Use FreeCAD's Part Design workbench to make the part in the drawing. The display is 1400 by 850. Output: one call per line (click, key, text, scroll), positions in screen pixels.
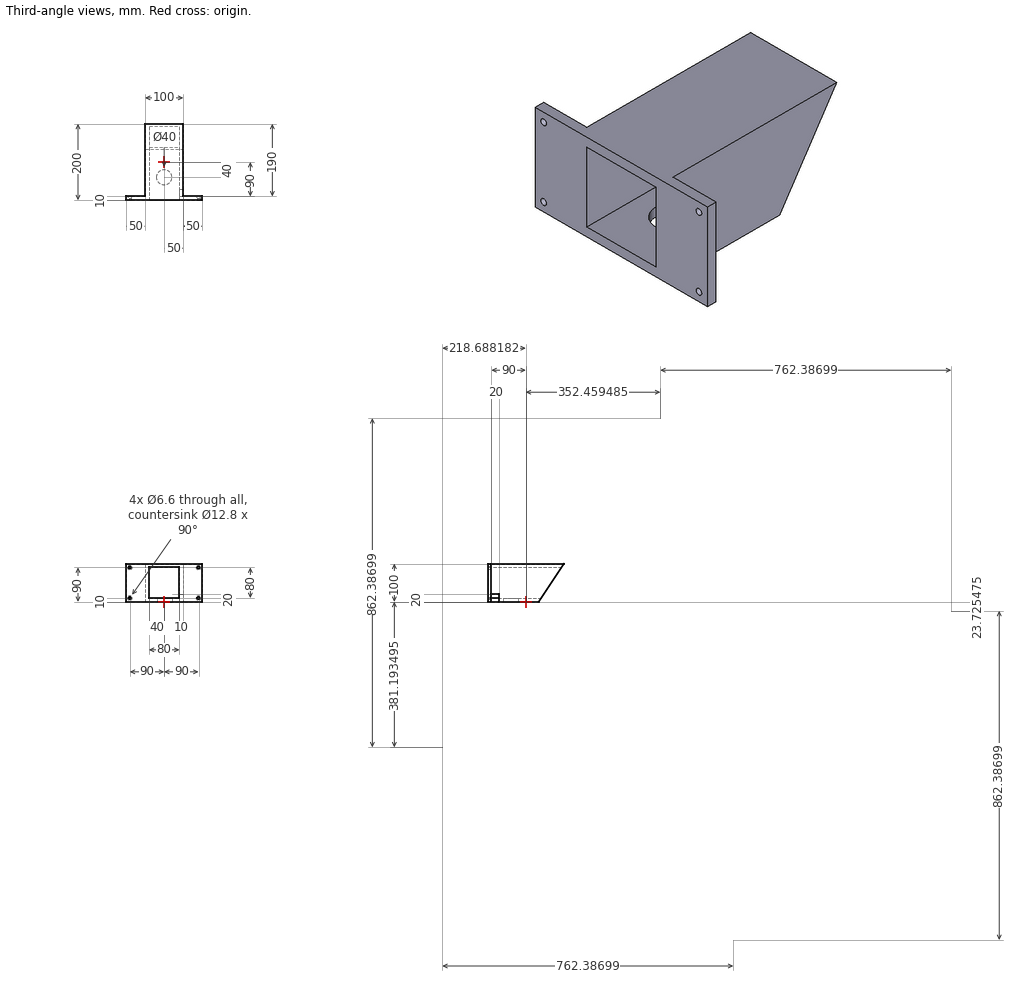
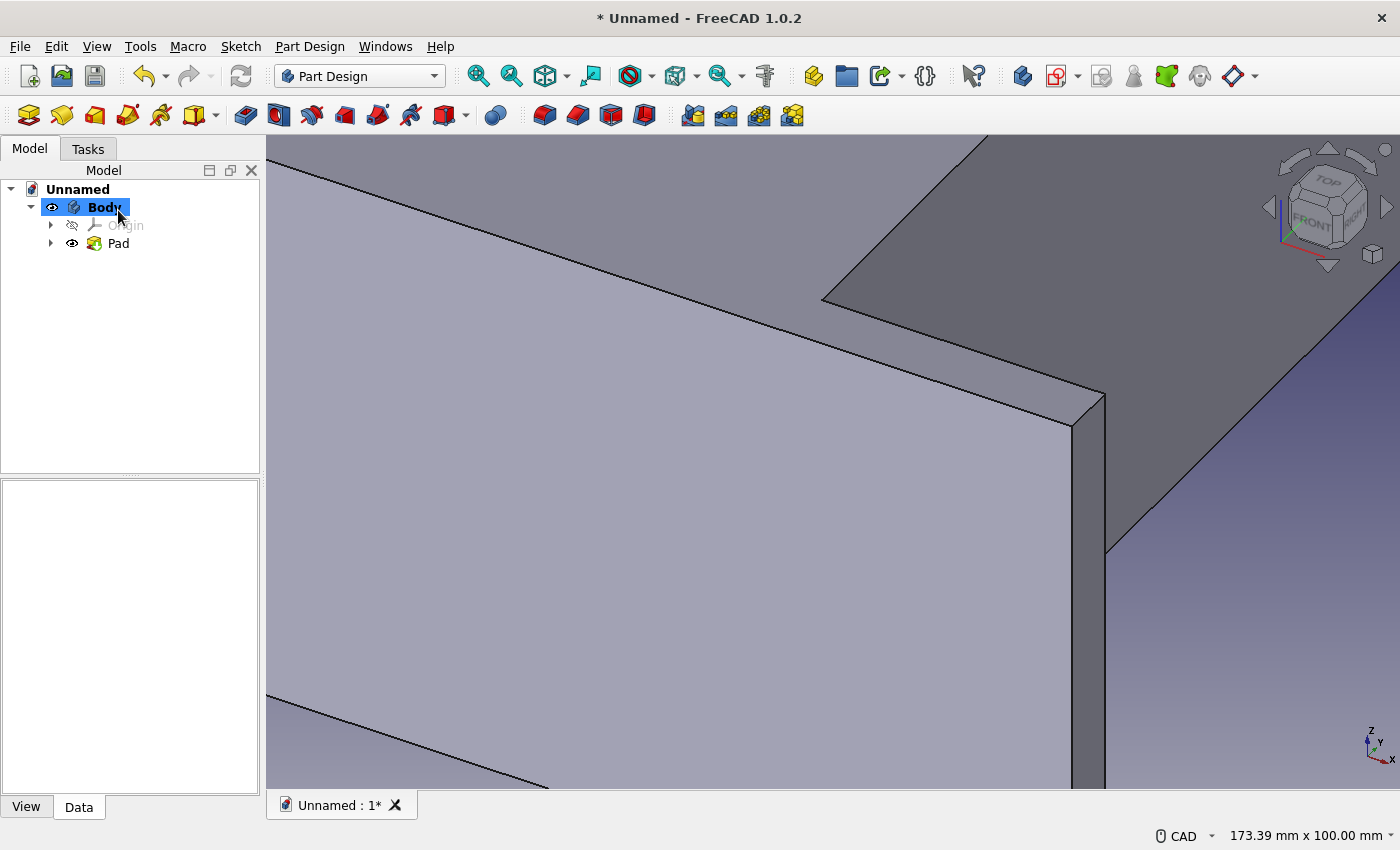
key(v)
key(f)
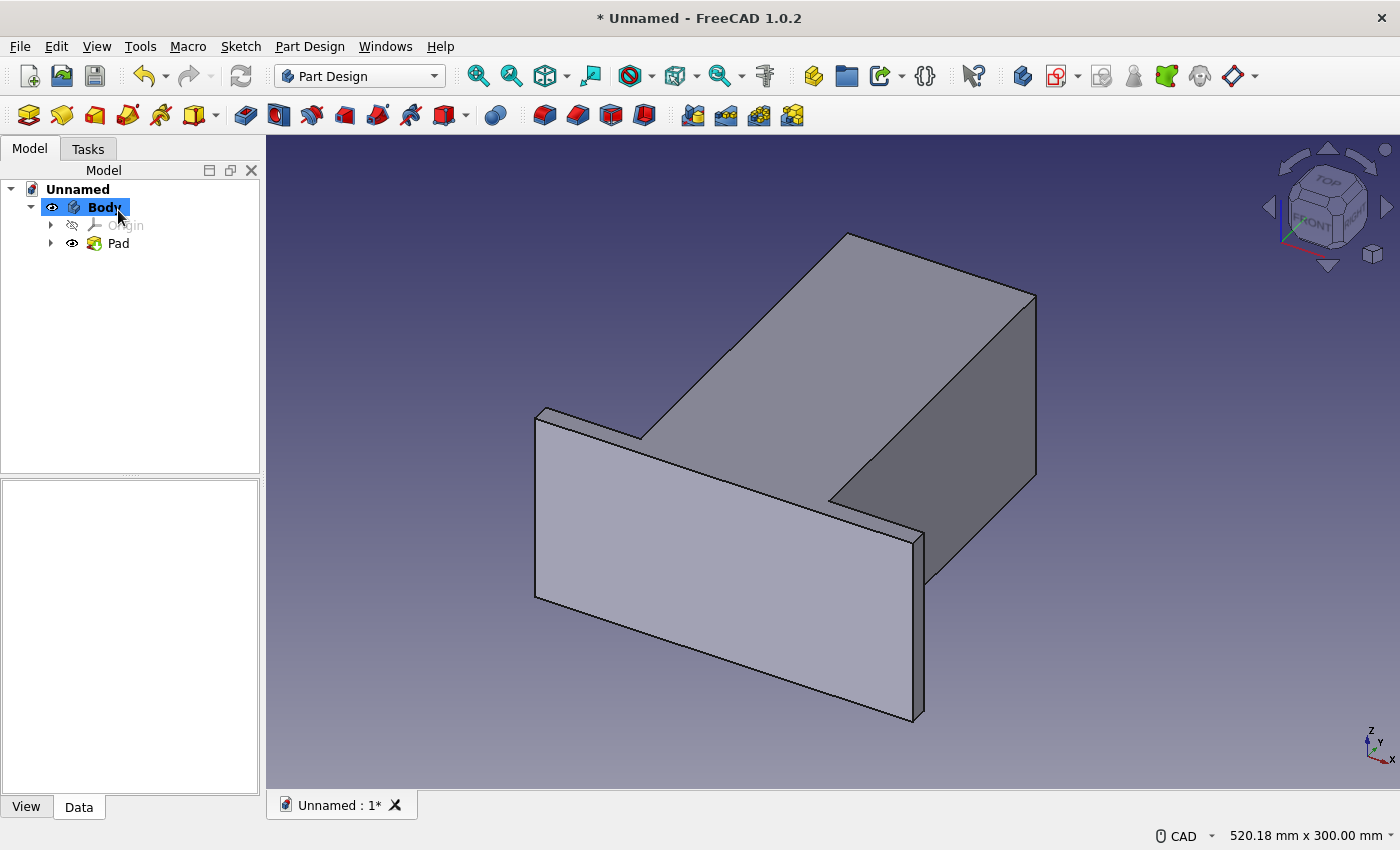
click(1056, 76)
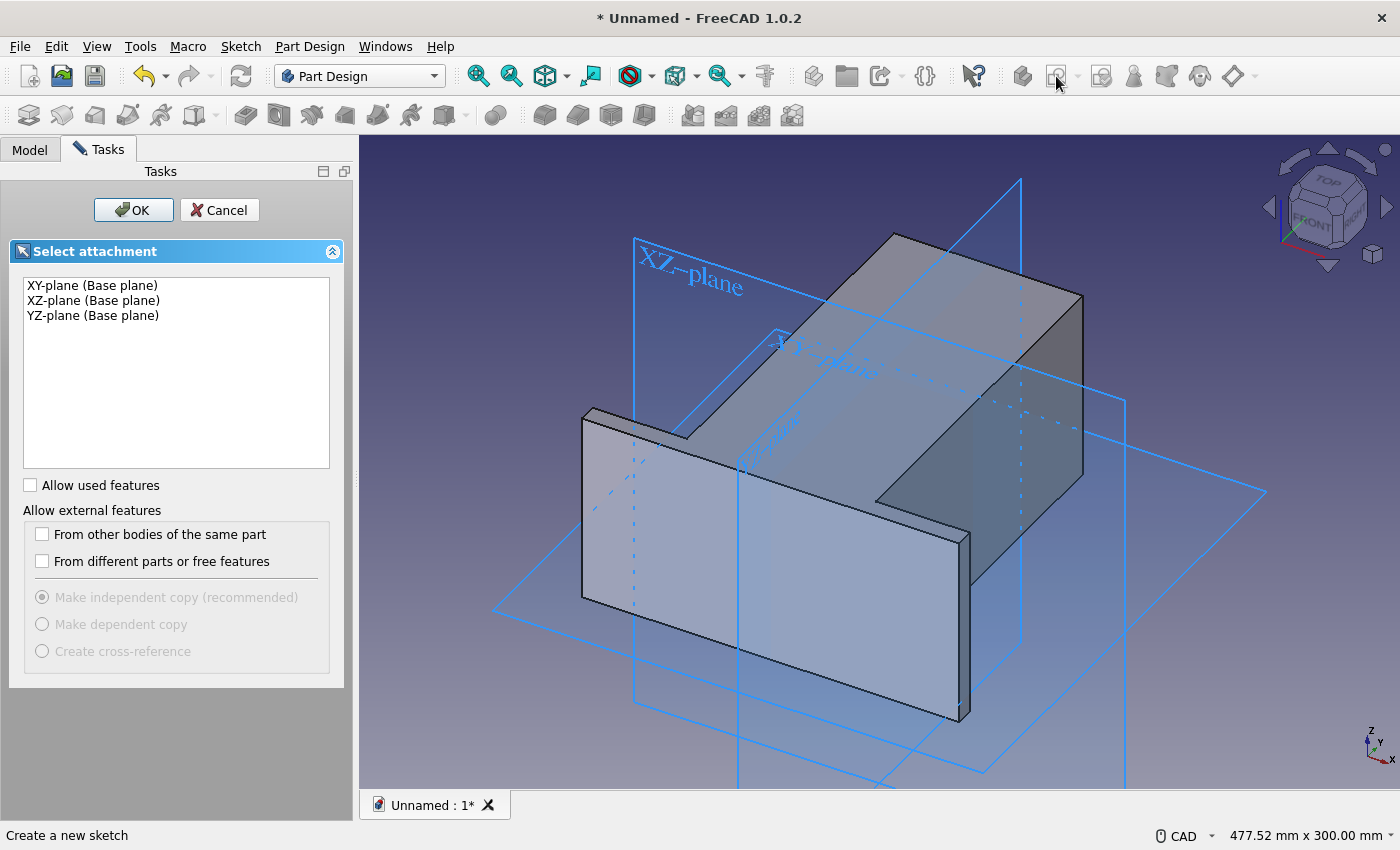
click(84, 316)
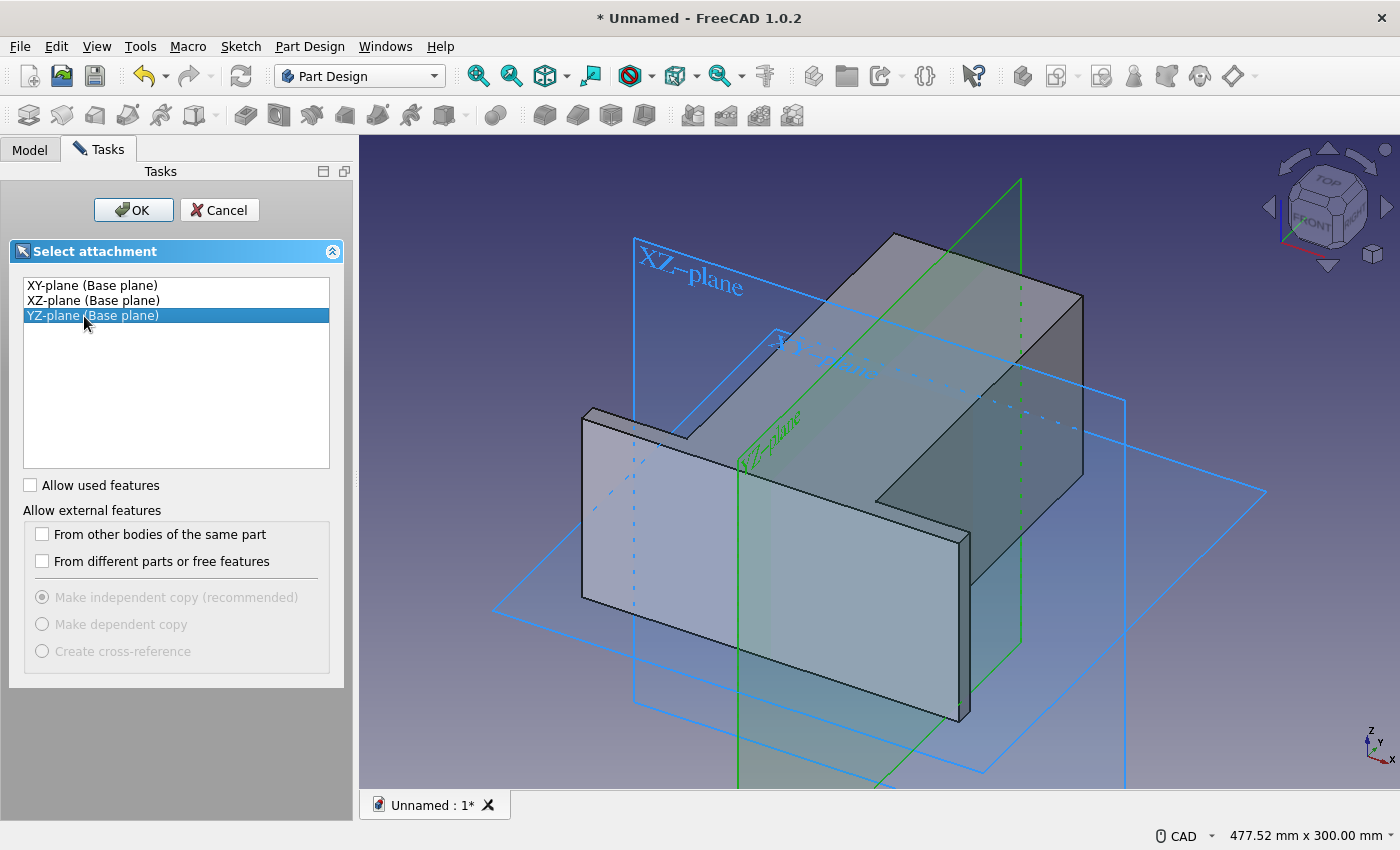
click(134, 210)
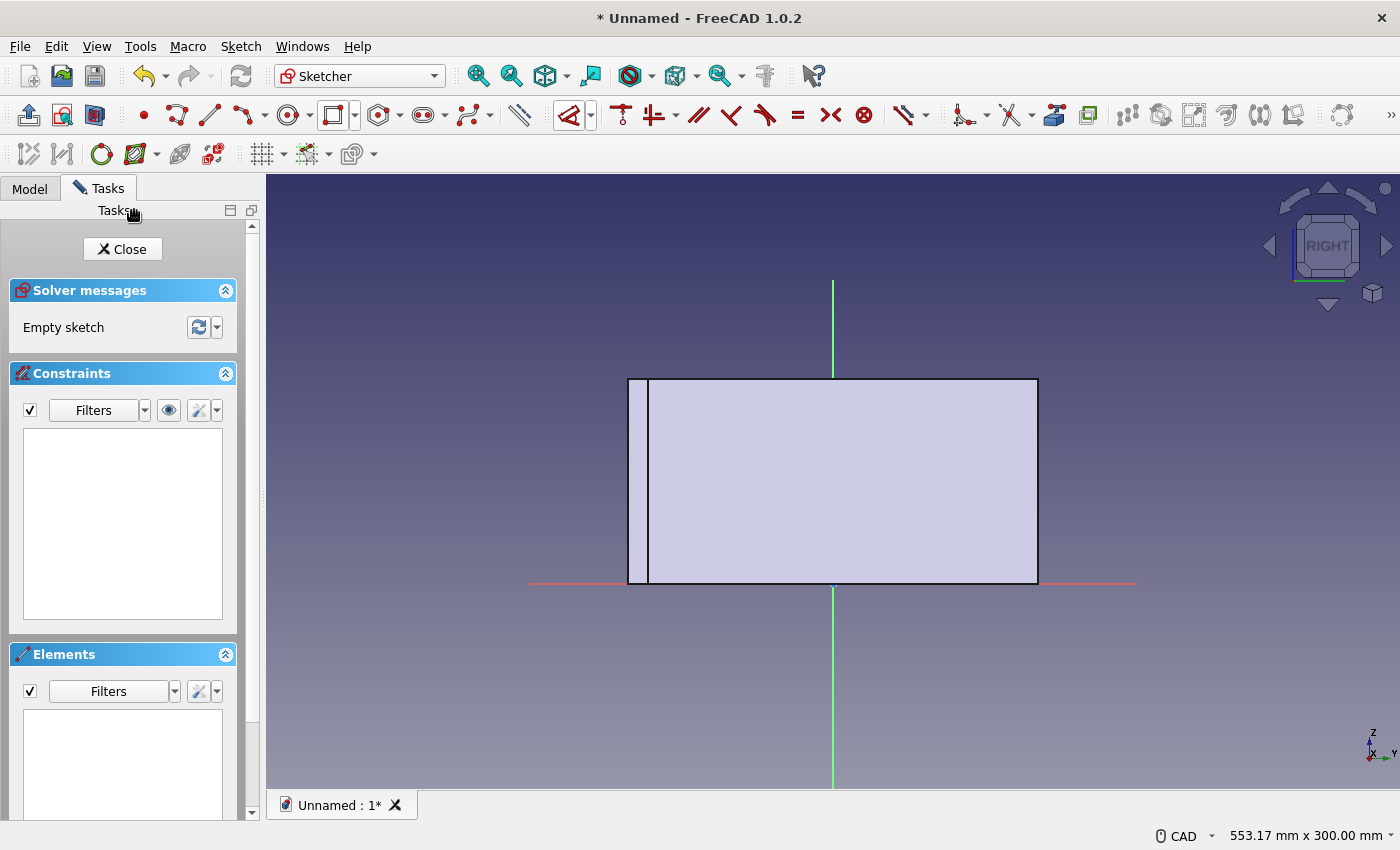
key(q)
key(s)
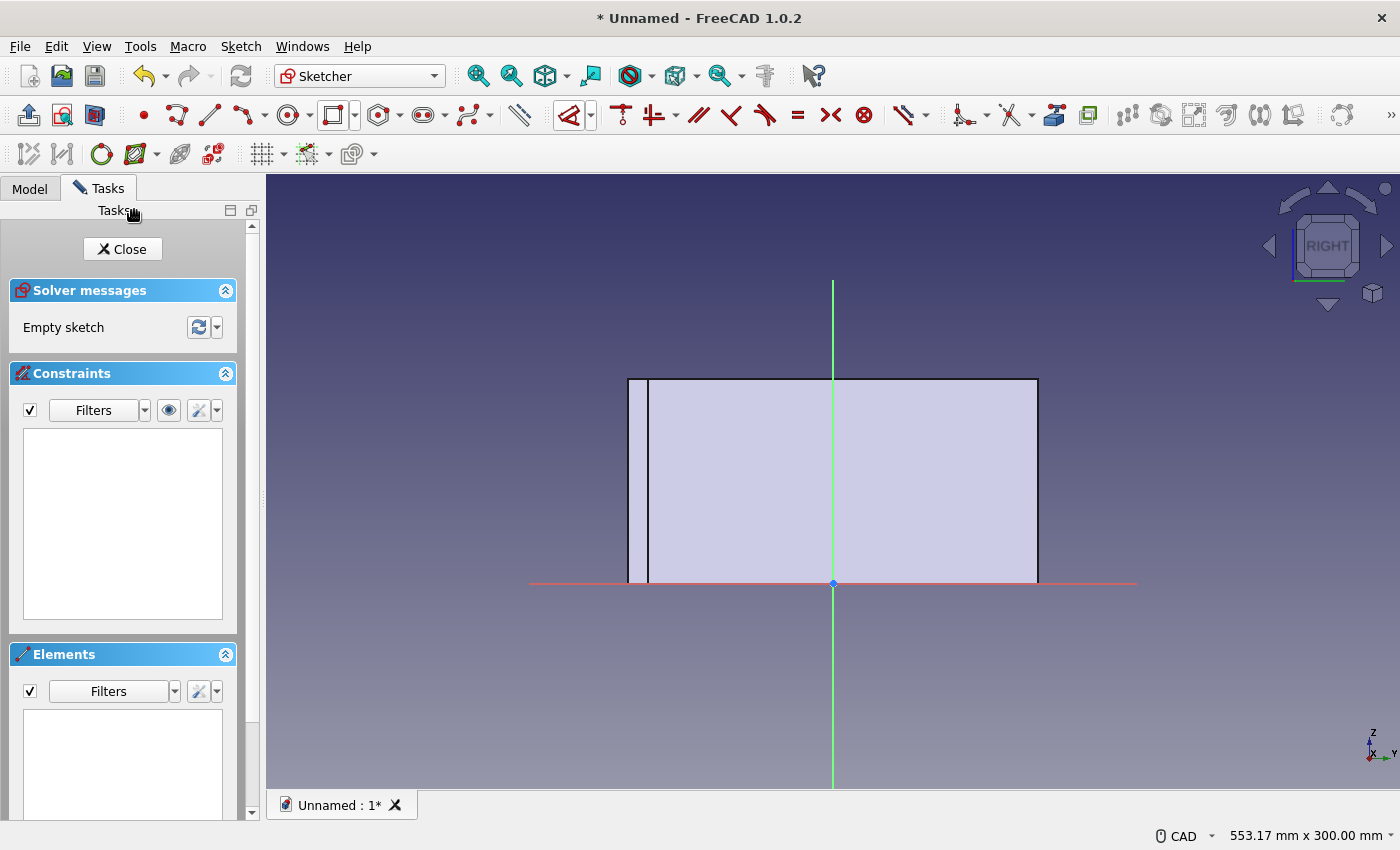
scroll(610, 400, down, 10)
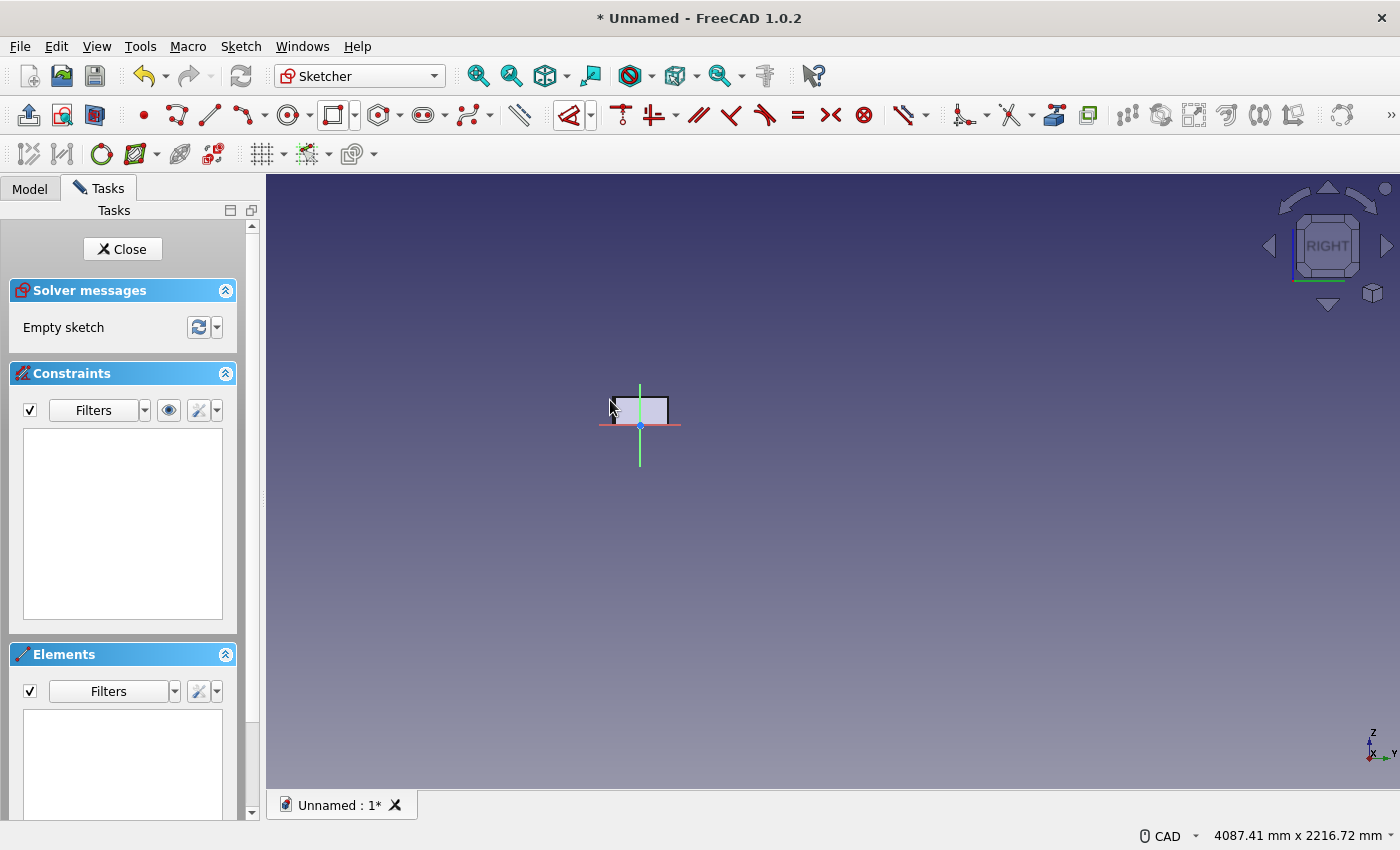
key(g)
key(m)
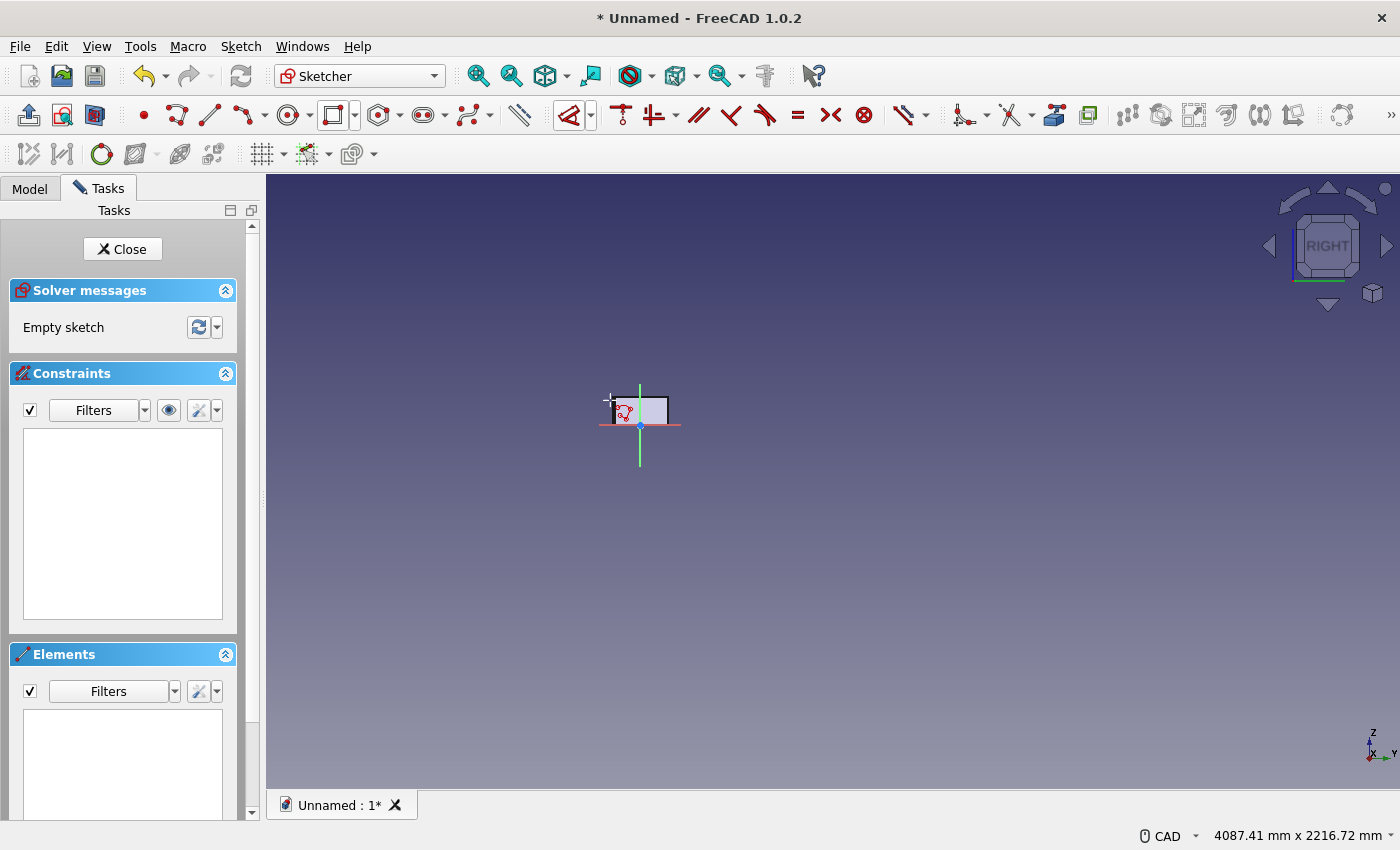
click(580, 531)
click(791, 671)